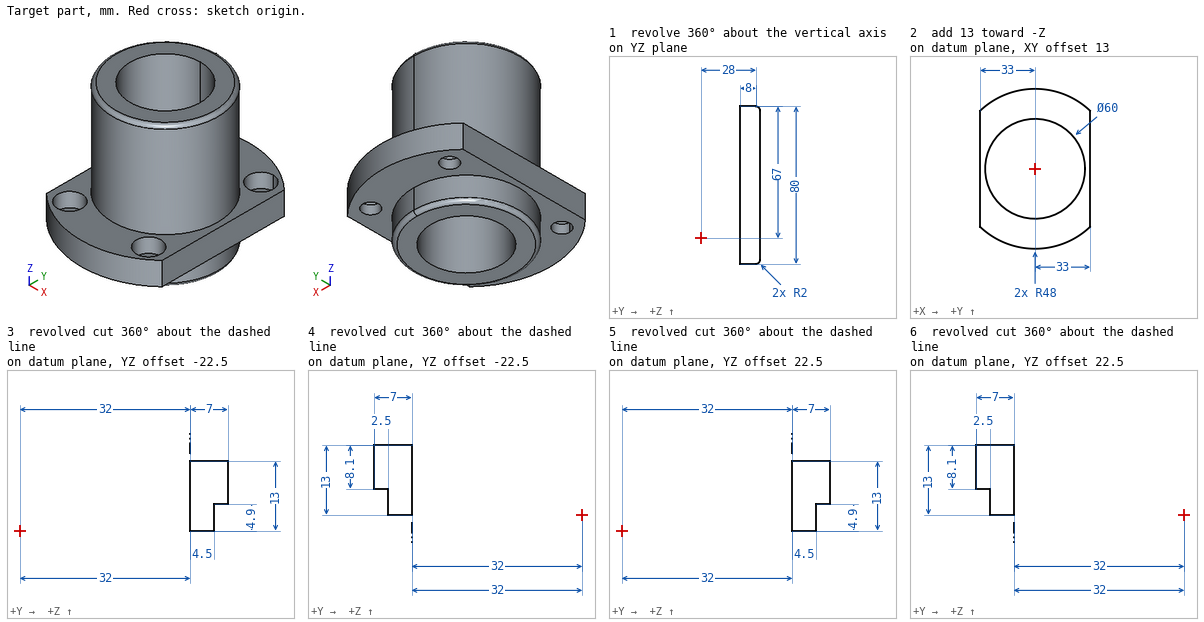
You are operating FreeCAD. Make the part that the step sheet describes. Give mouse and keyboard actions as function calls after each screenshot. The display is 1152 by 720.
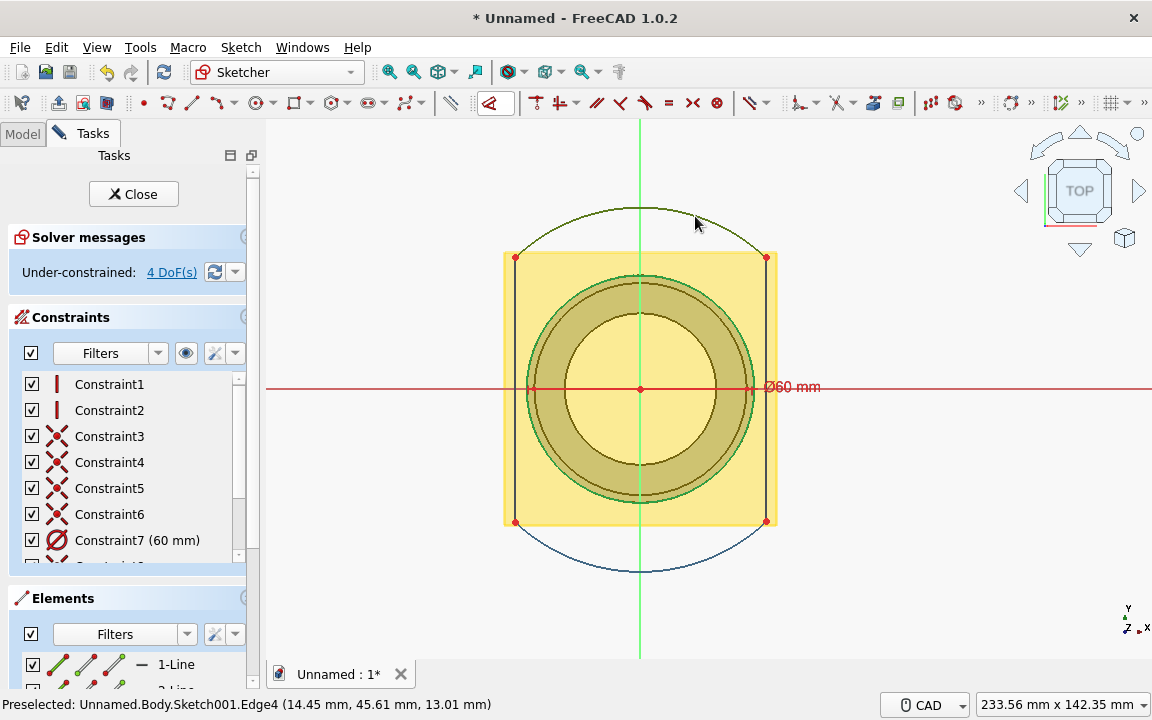
click(670, 104)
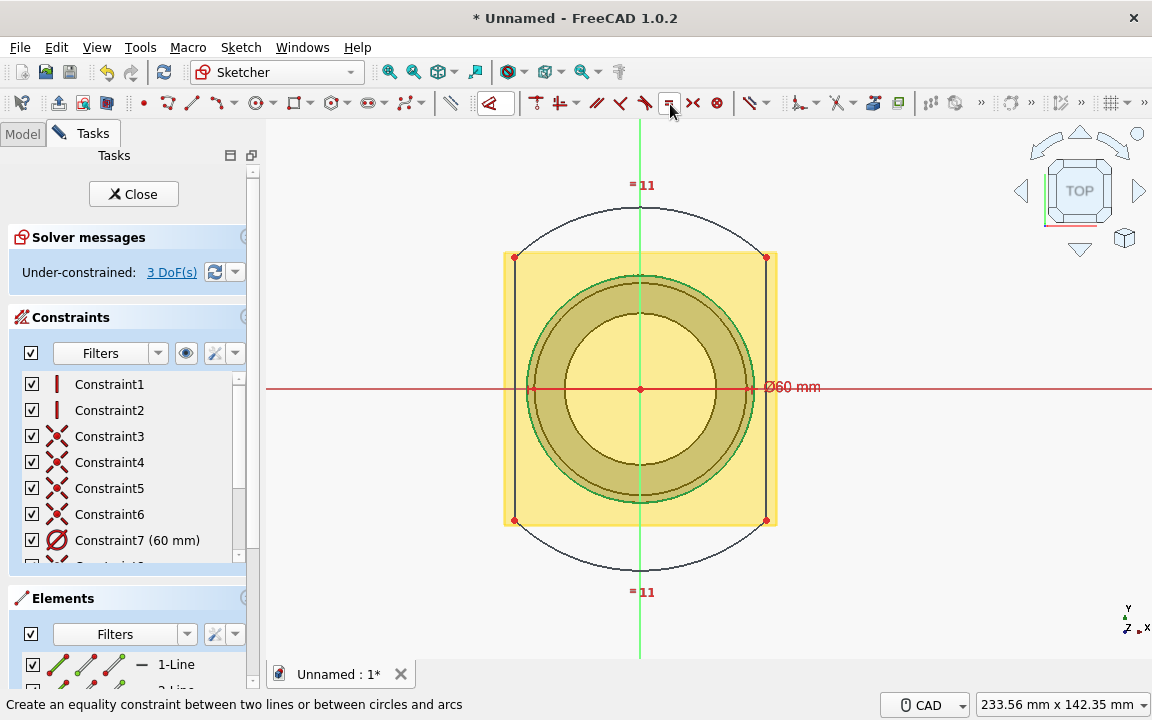
click(586, 562)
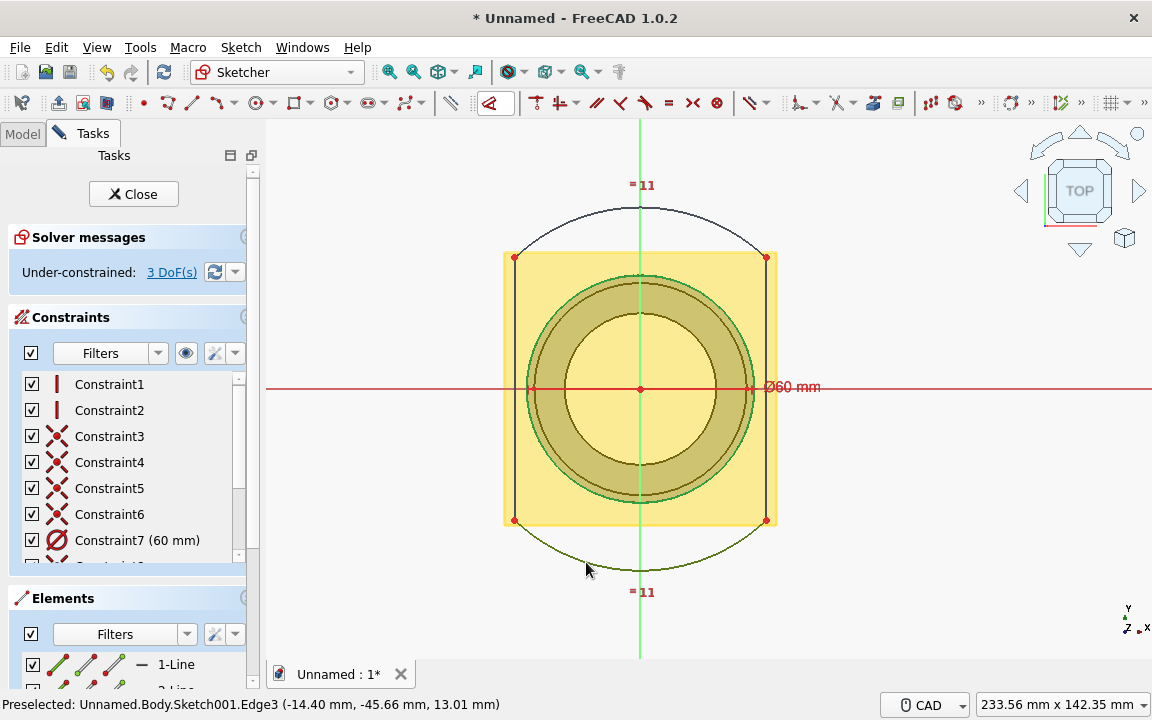
key(k)
key(r)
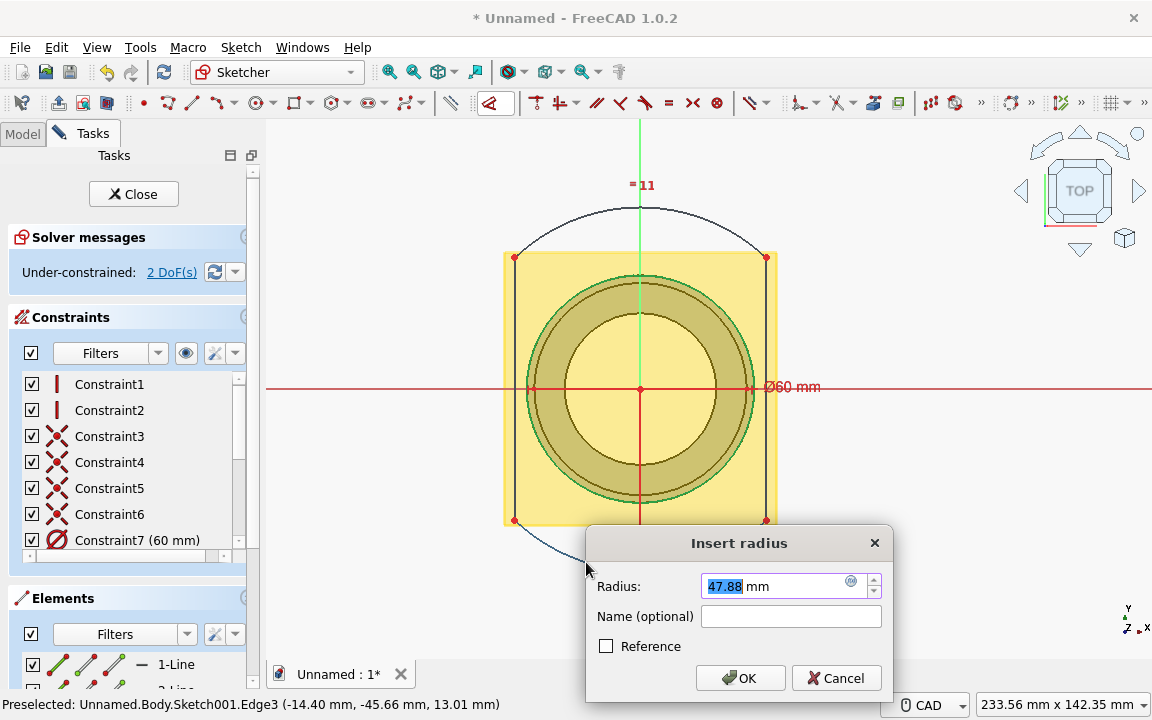
text(48)
key(Return)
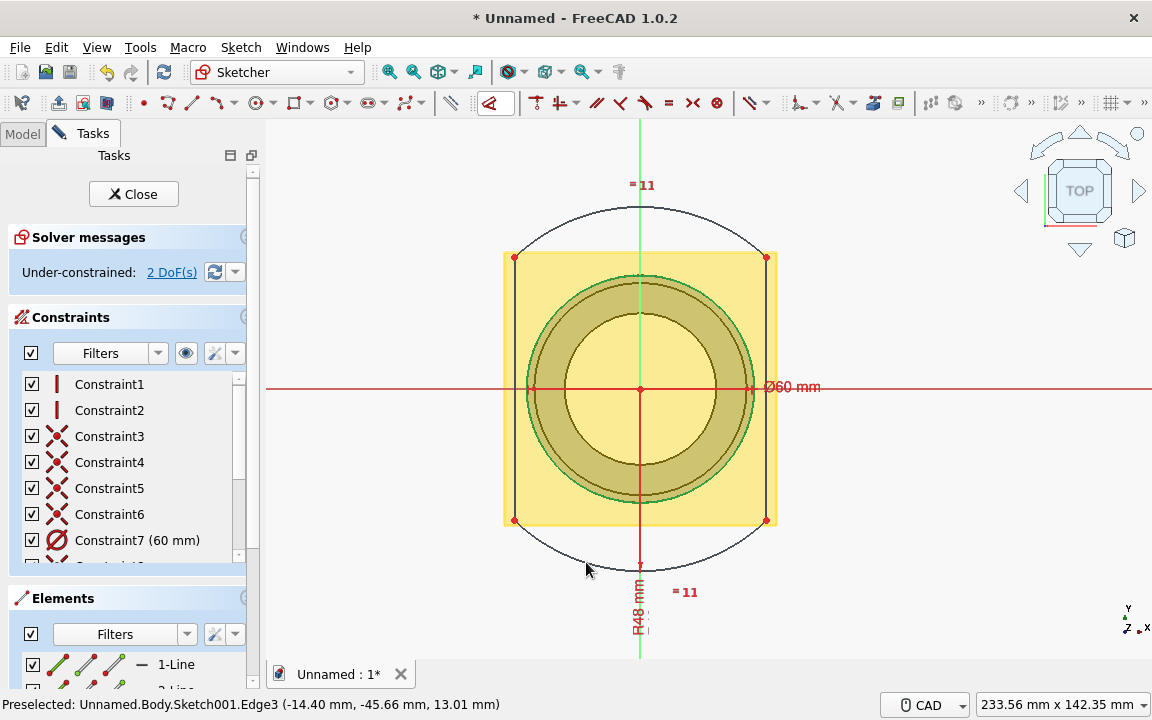
click(515, 257)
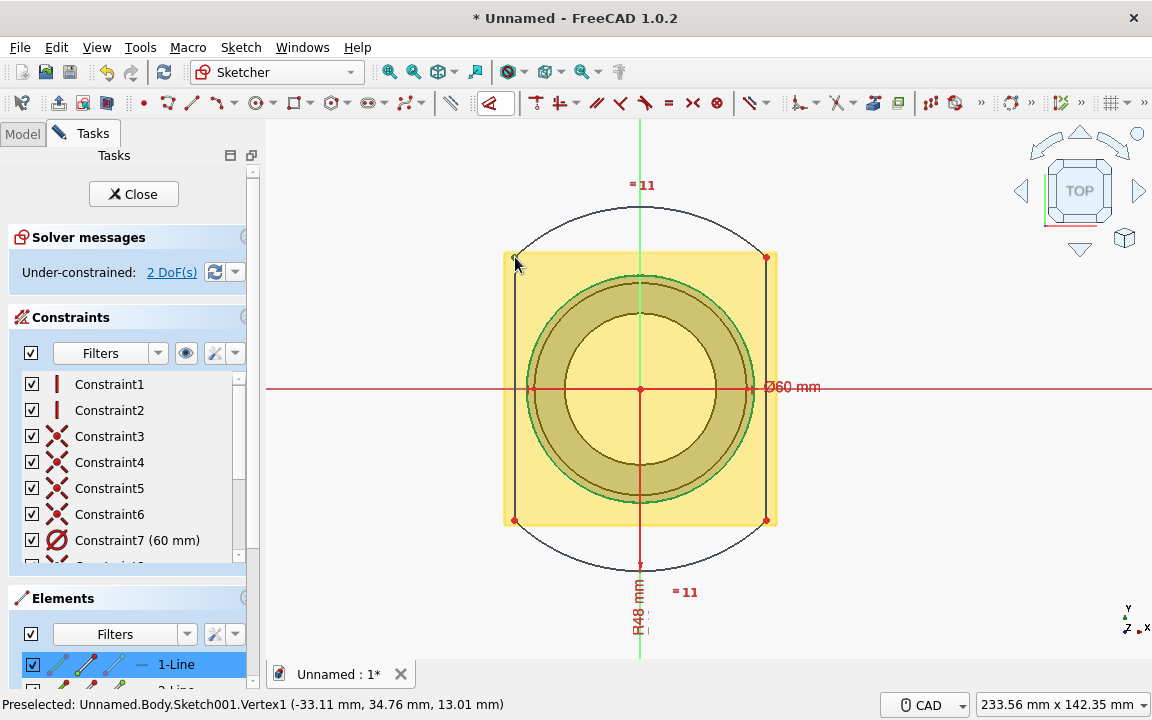
click(508, 104)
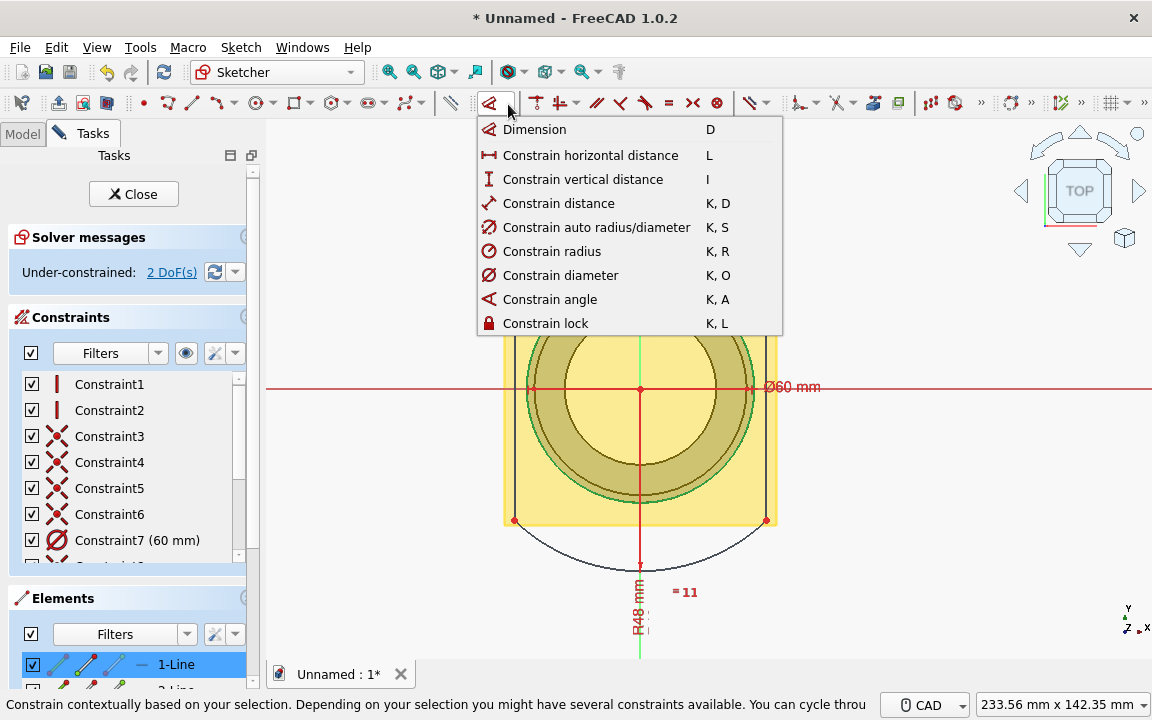
click(630, 155)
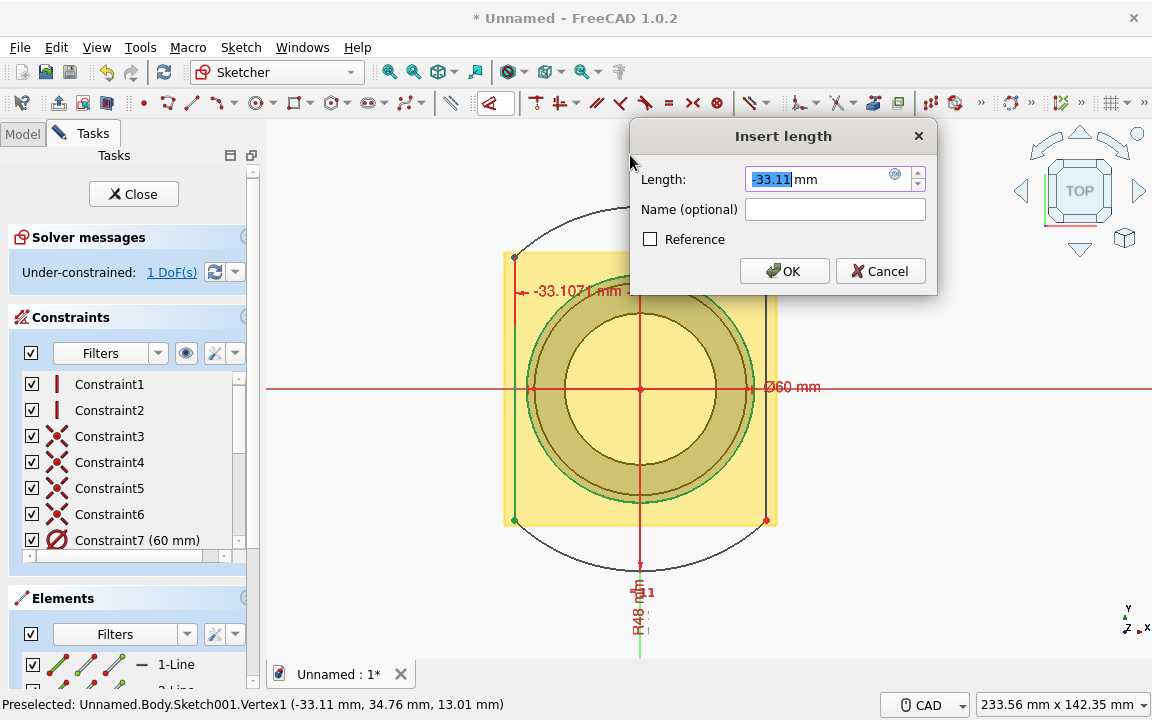
text(-33)
key(Return)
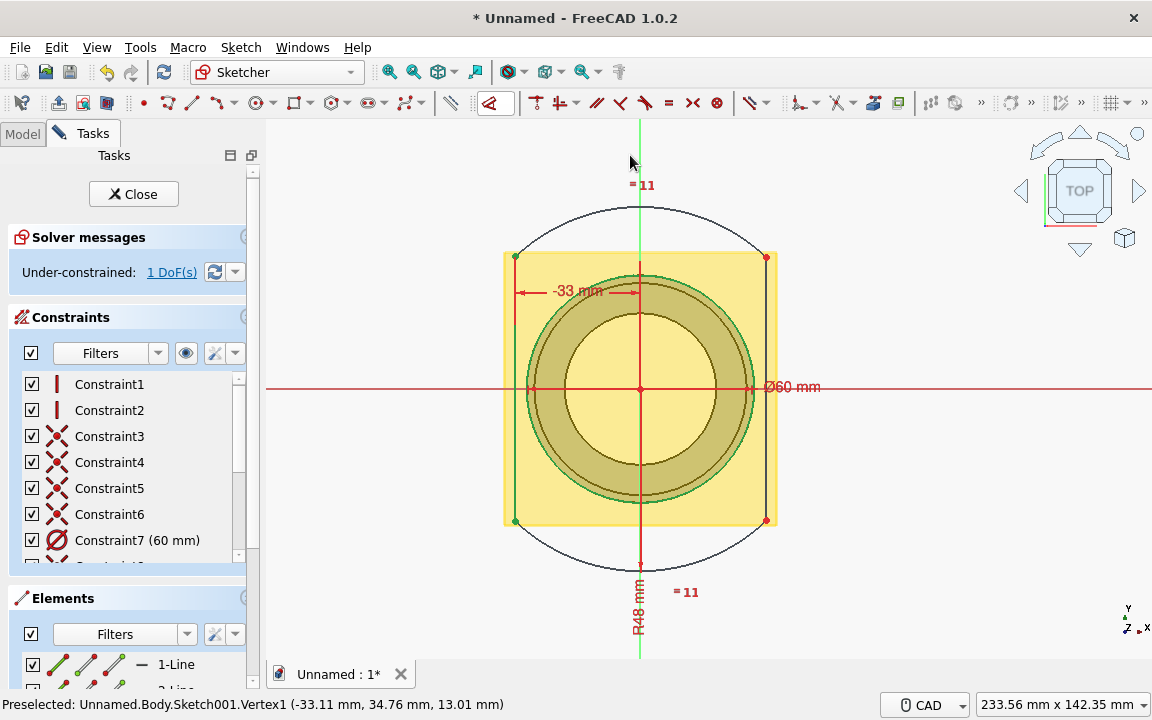
click(766, 521)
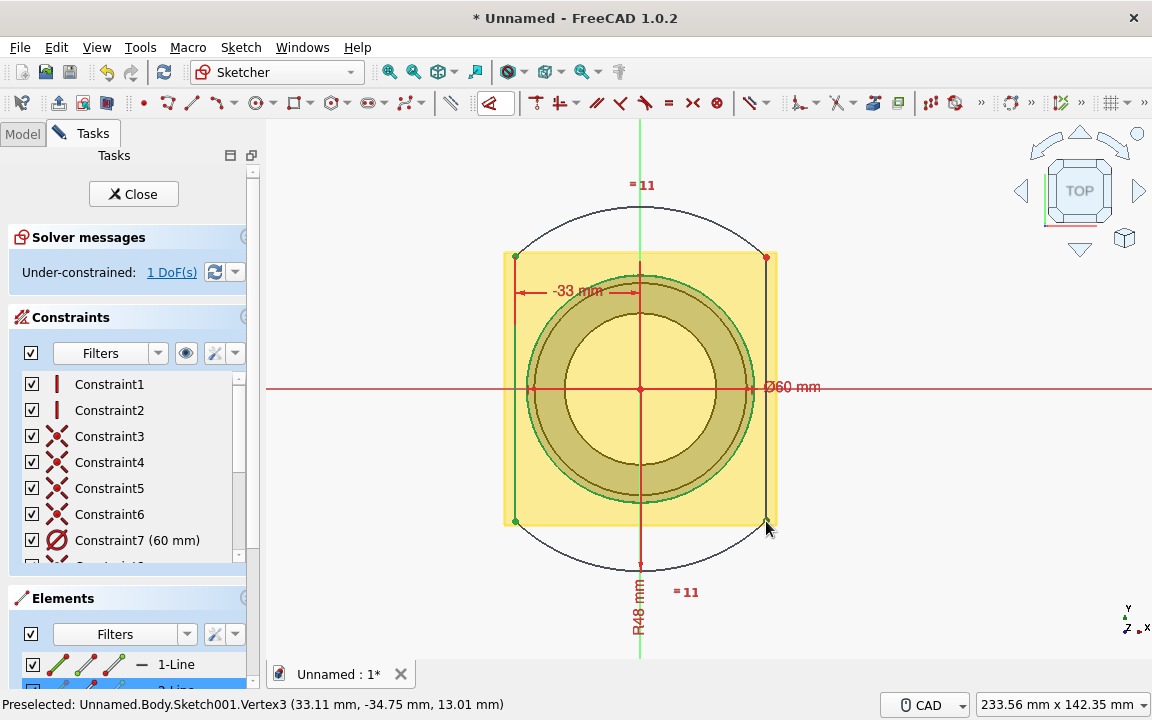
click(508, 104)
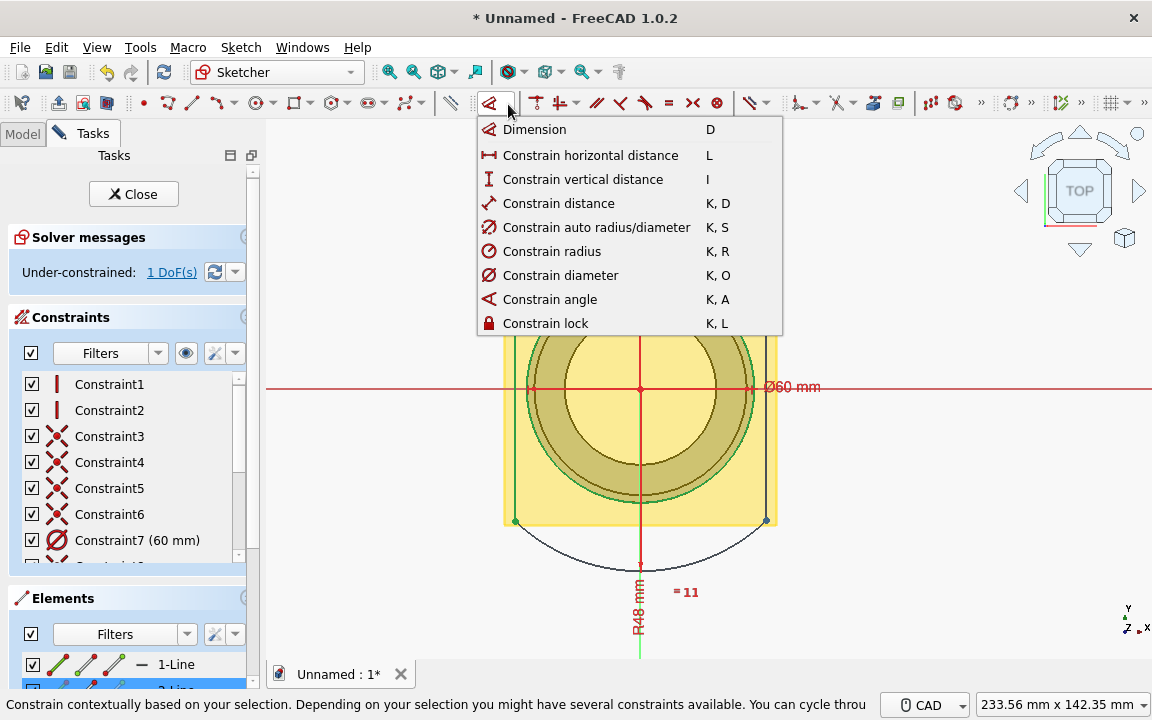
click(630, 155)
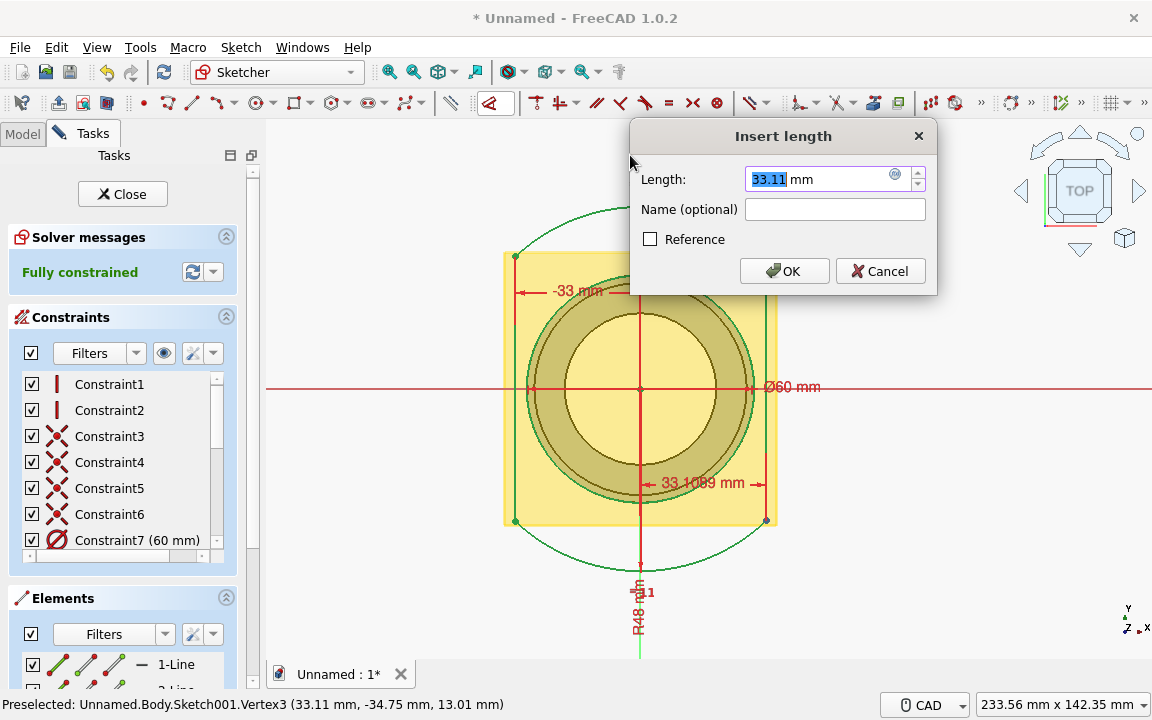
text(33)
key(Return)